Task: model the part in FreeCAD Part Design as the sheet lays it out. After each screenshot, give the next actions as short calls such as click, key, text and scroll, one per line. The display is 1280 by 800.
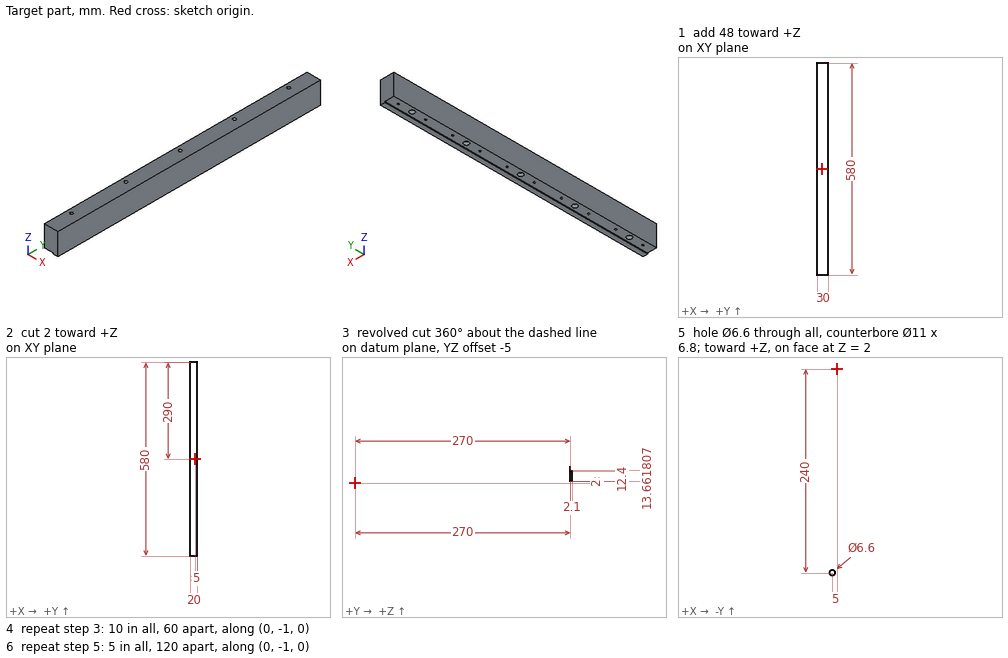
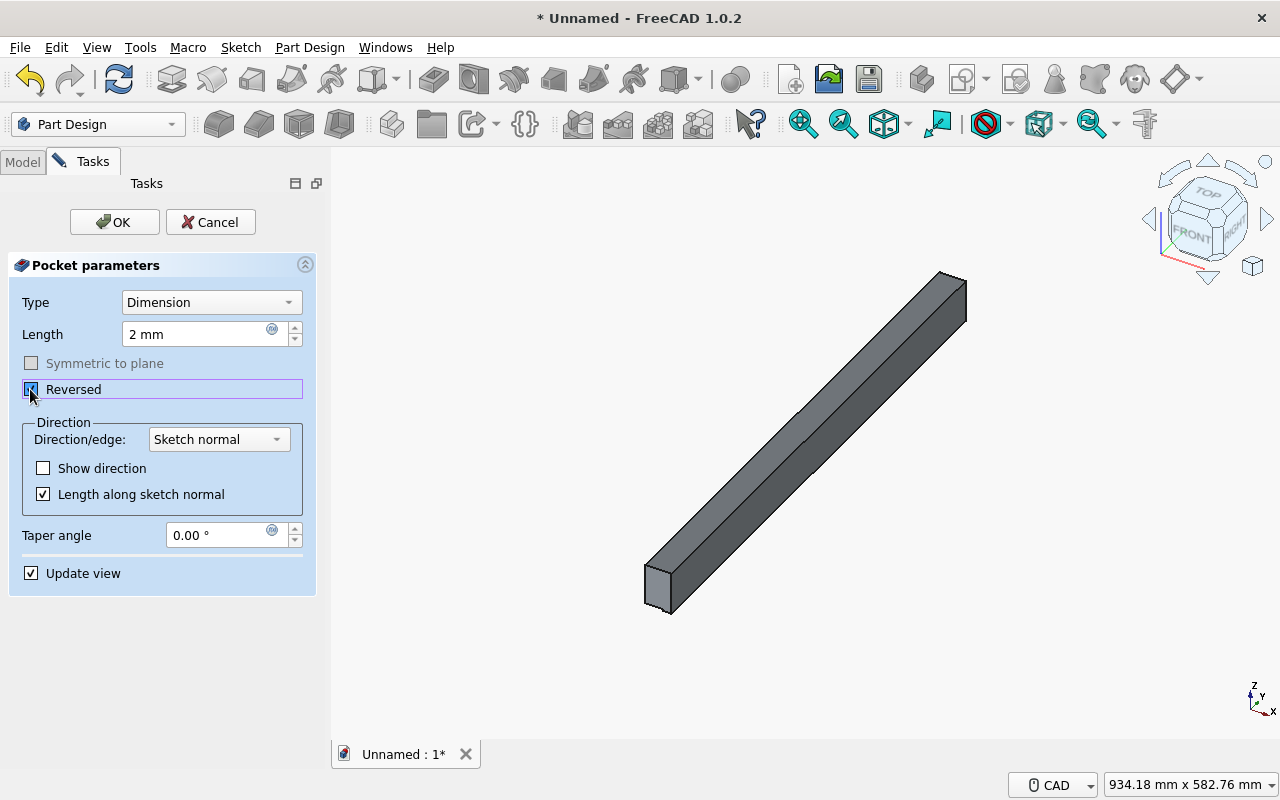
click(115, 222)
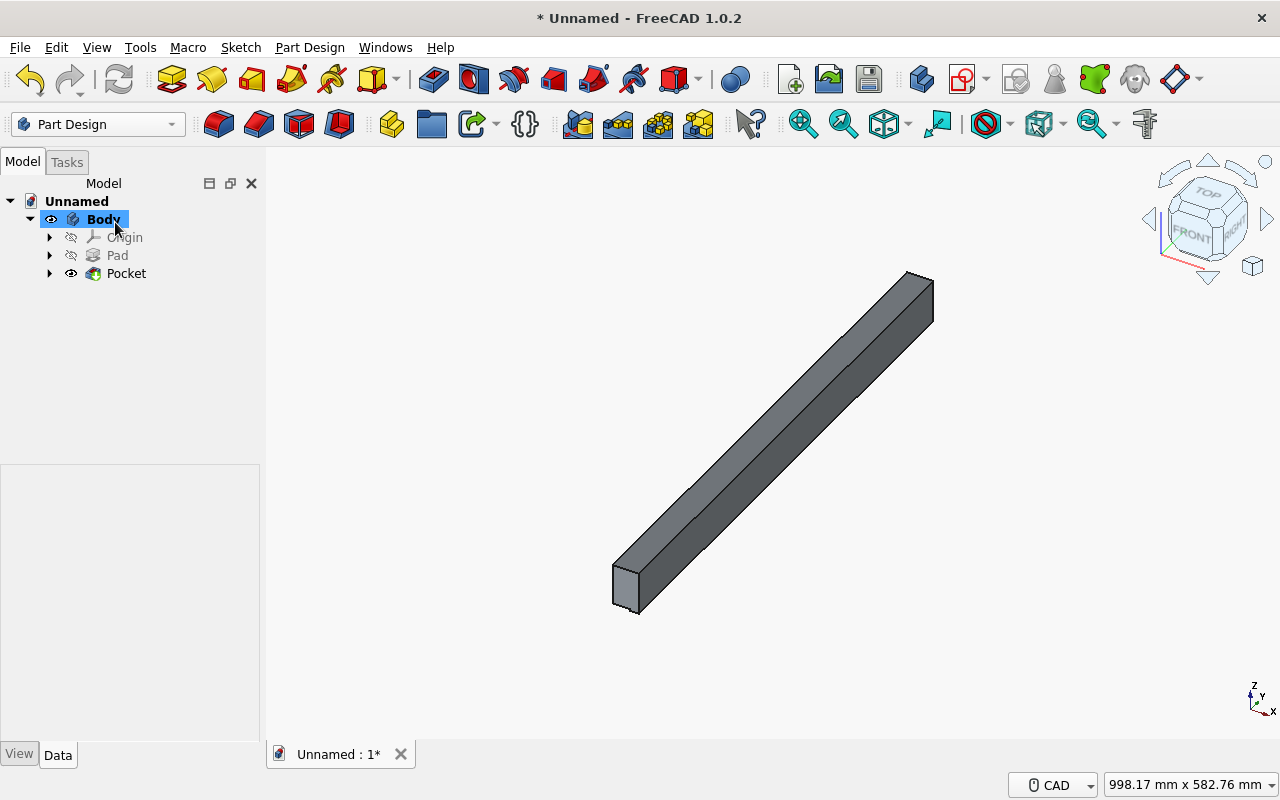
click(50, 237)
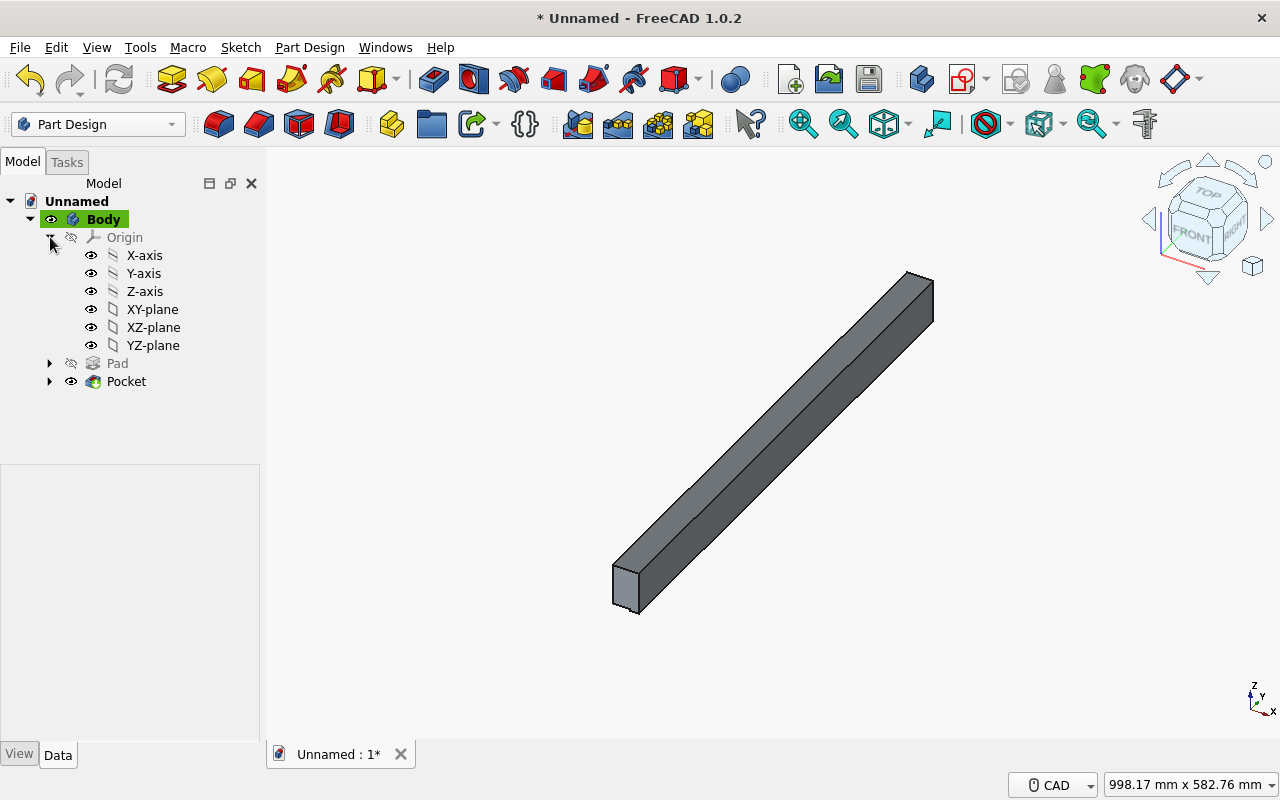
click(136, 345)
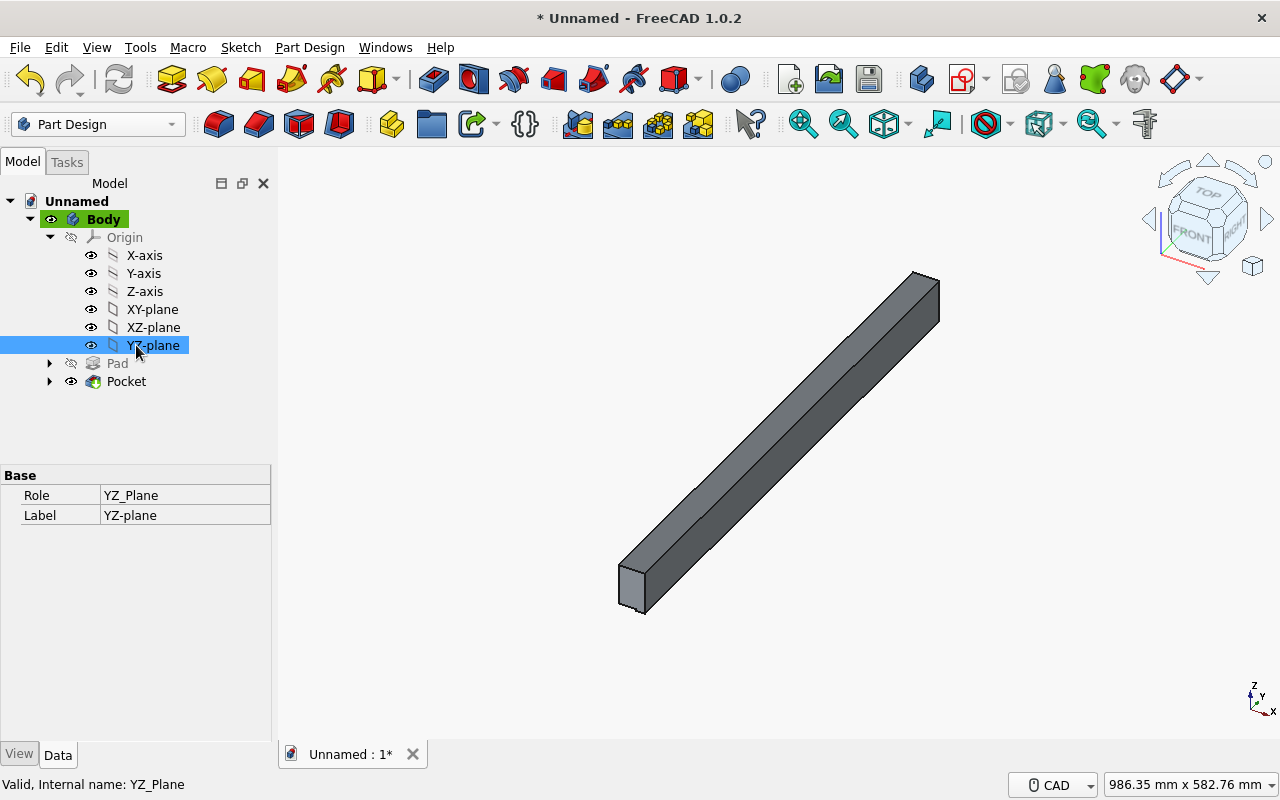
click(1176, 80)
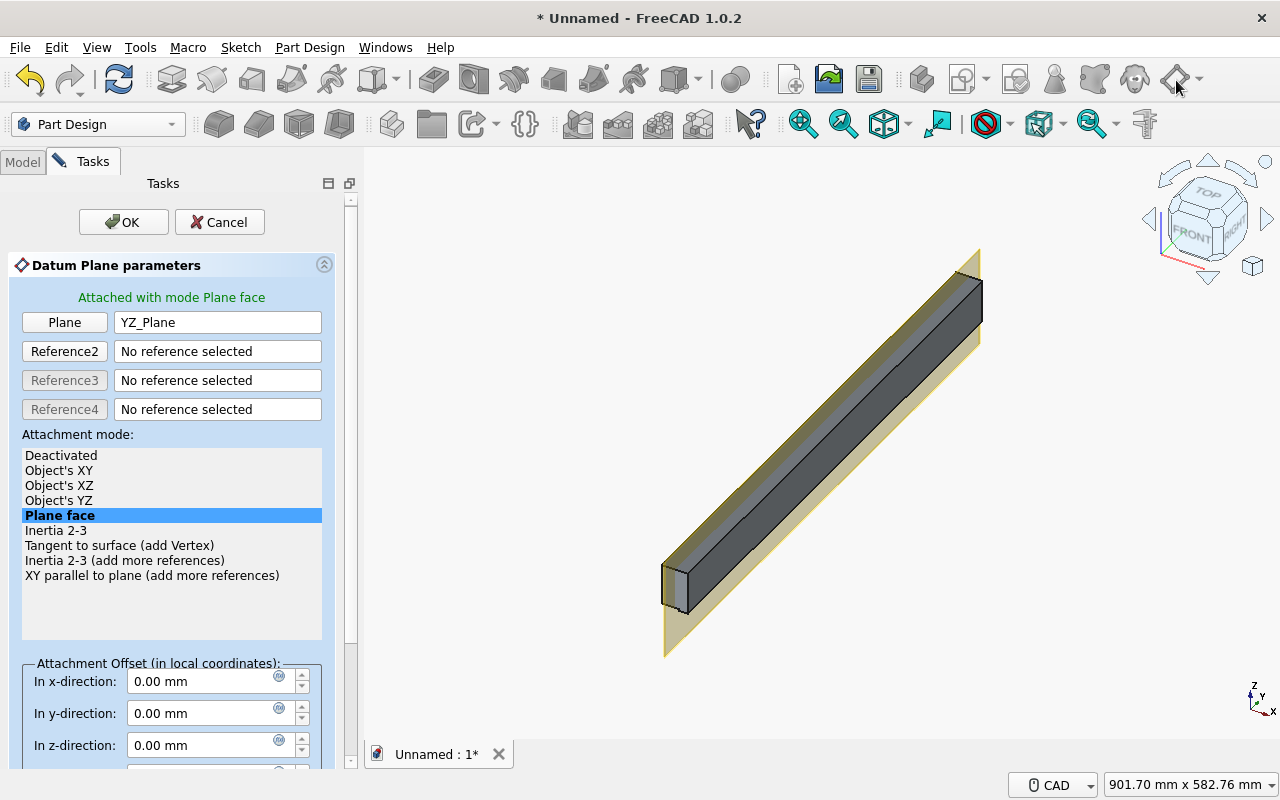
triple_click(210, 745)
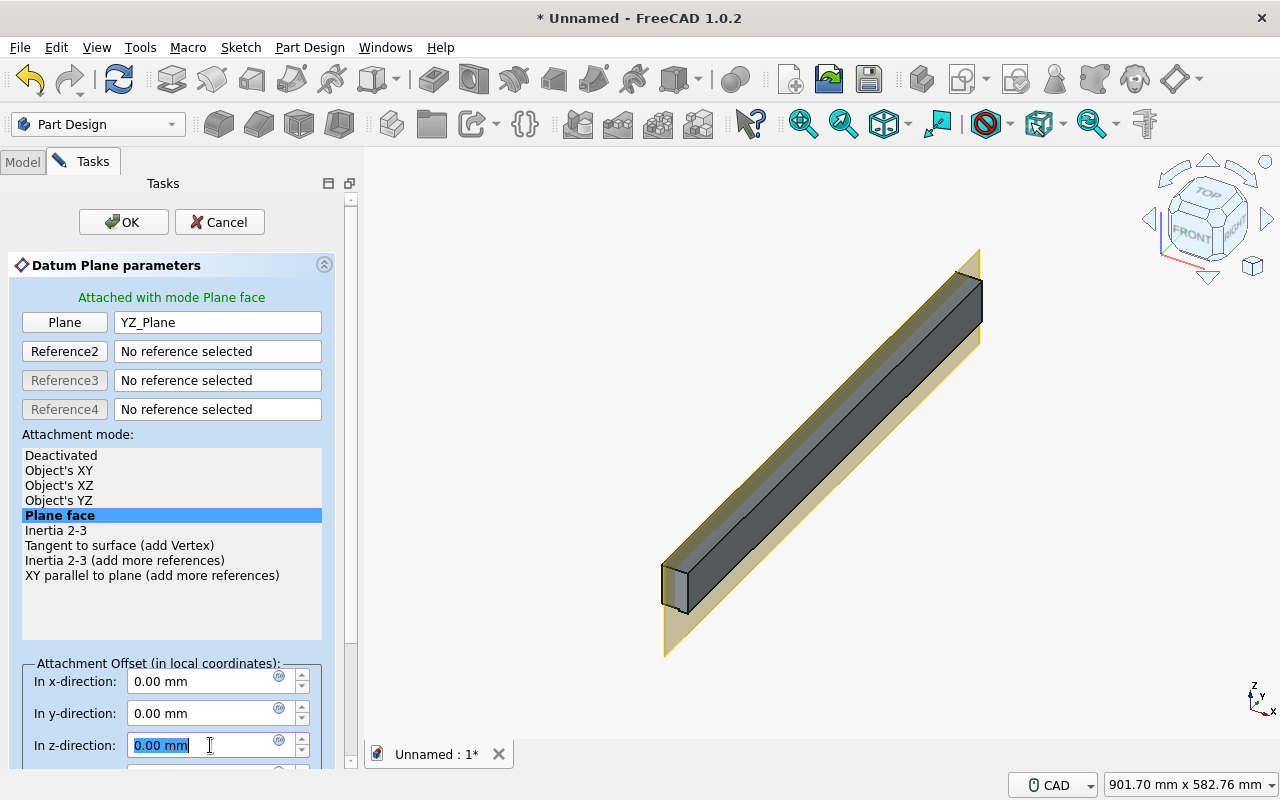
text(-5)
key(Tab)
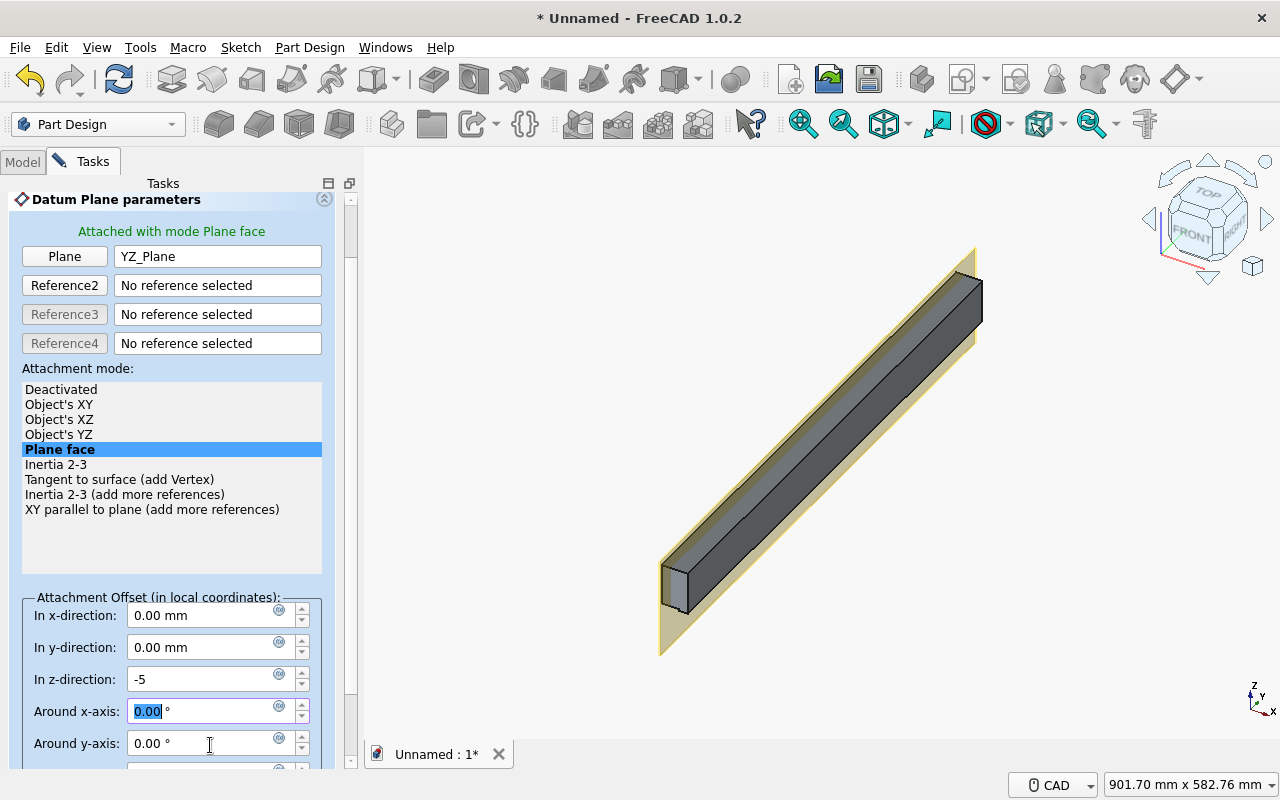
scroll(351, 480, up, 2)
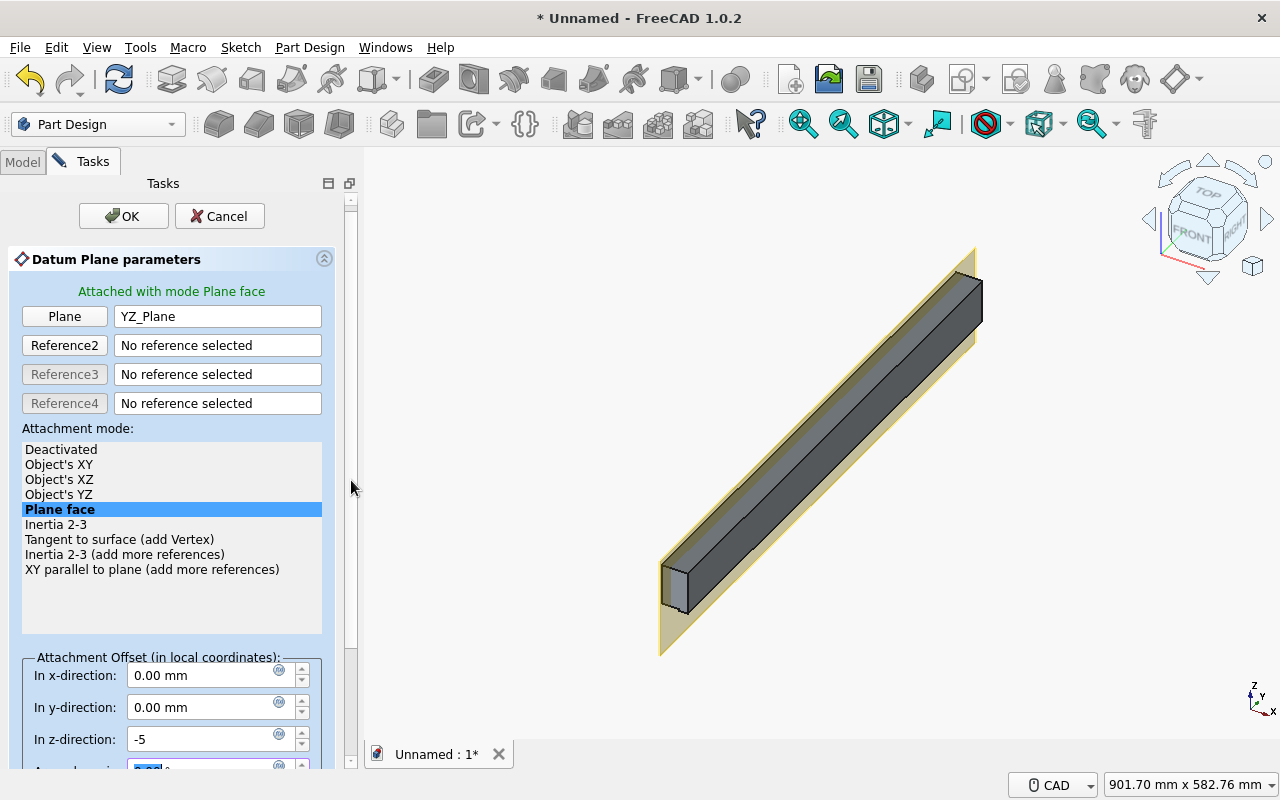
click(124, 222)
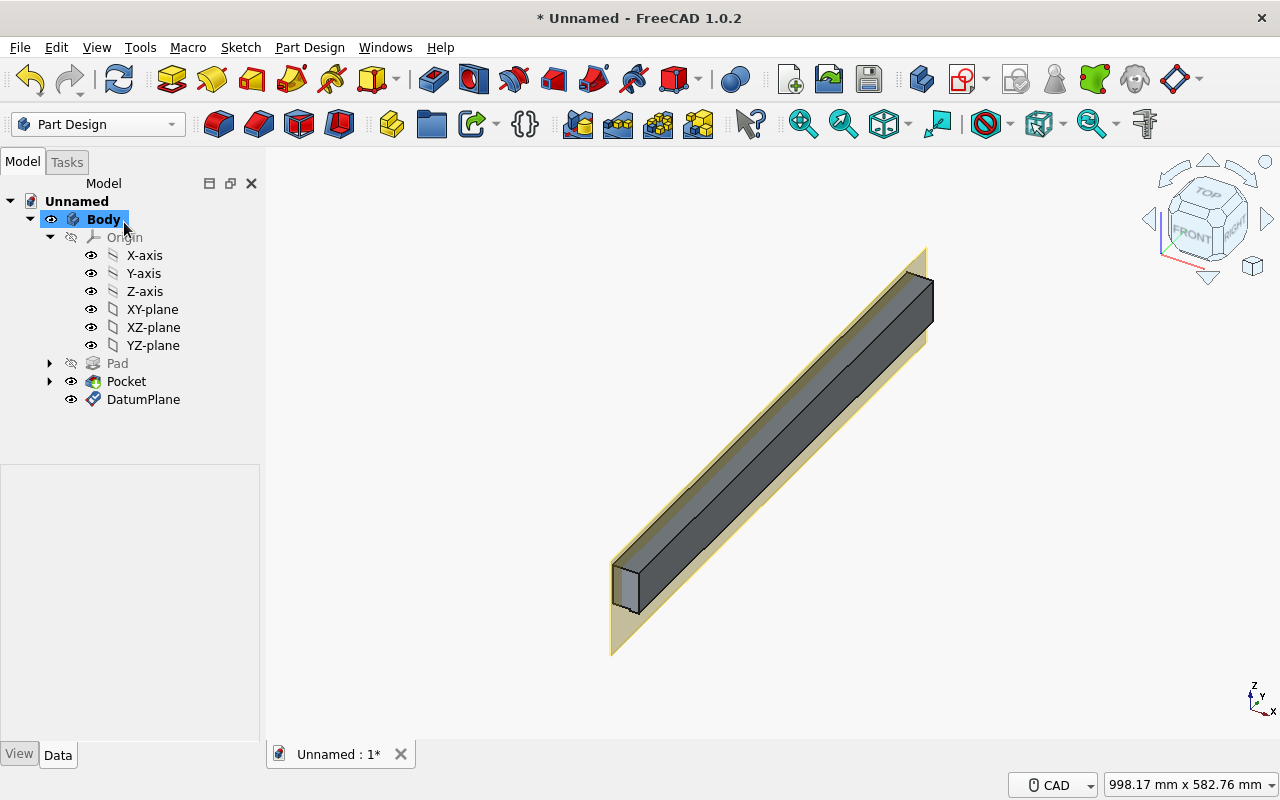
click(116, 399)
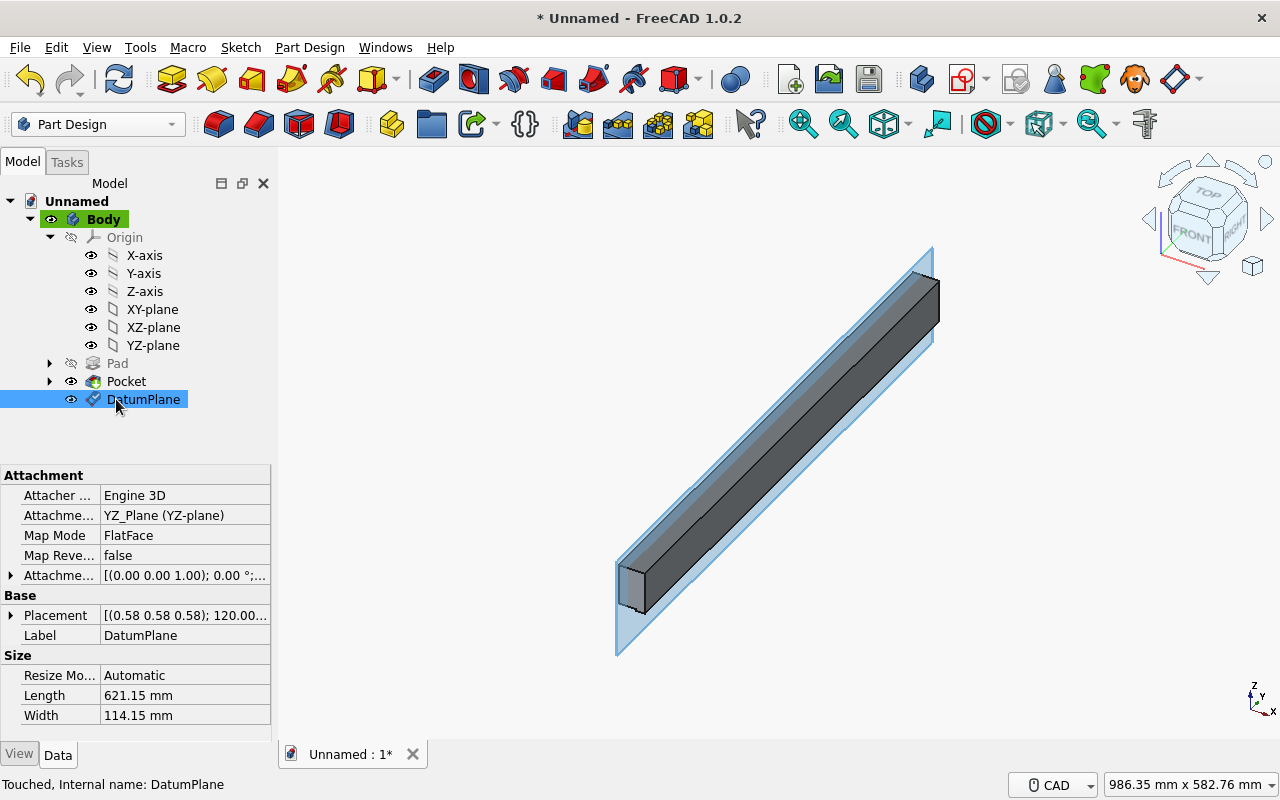
click(962, 80)